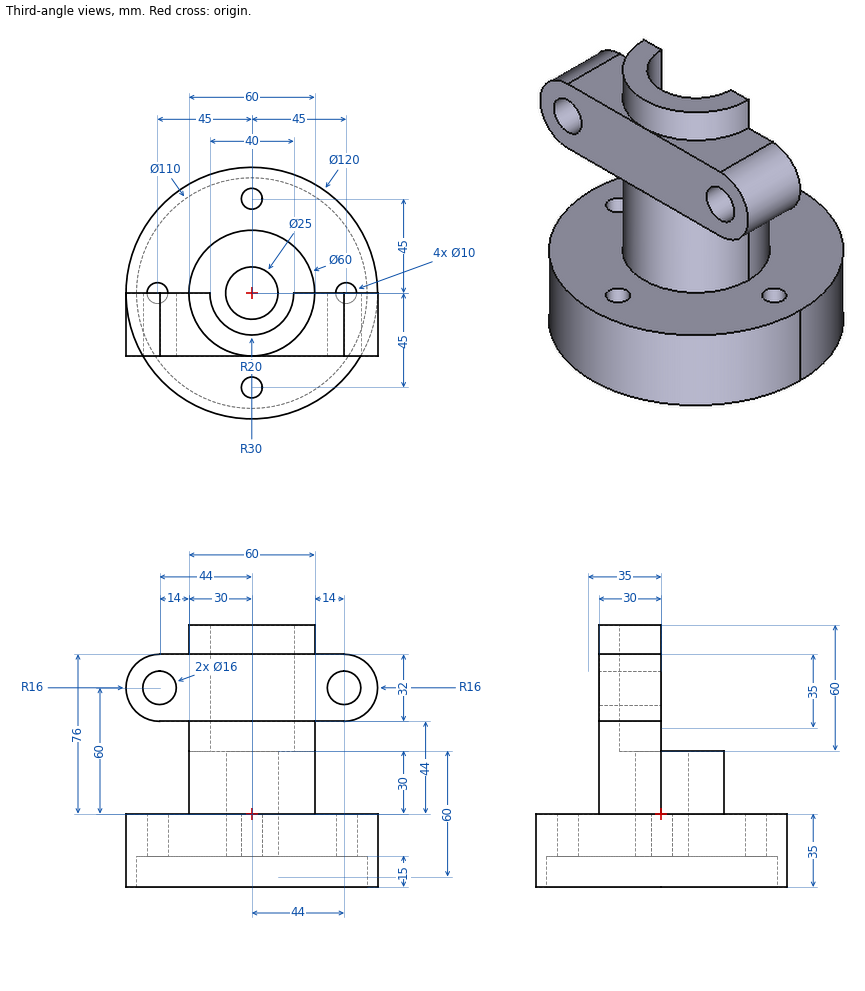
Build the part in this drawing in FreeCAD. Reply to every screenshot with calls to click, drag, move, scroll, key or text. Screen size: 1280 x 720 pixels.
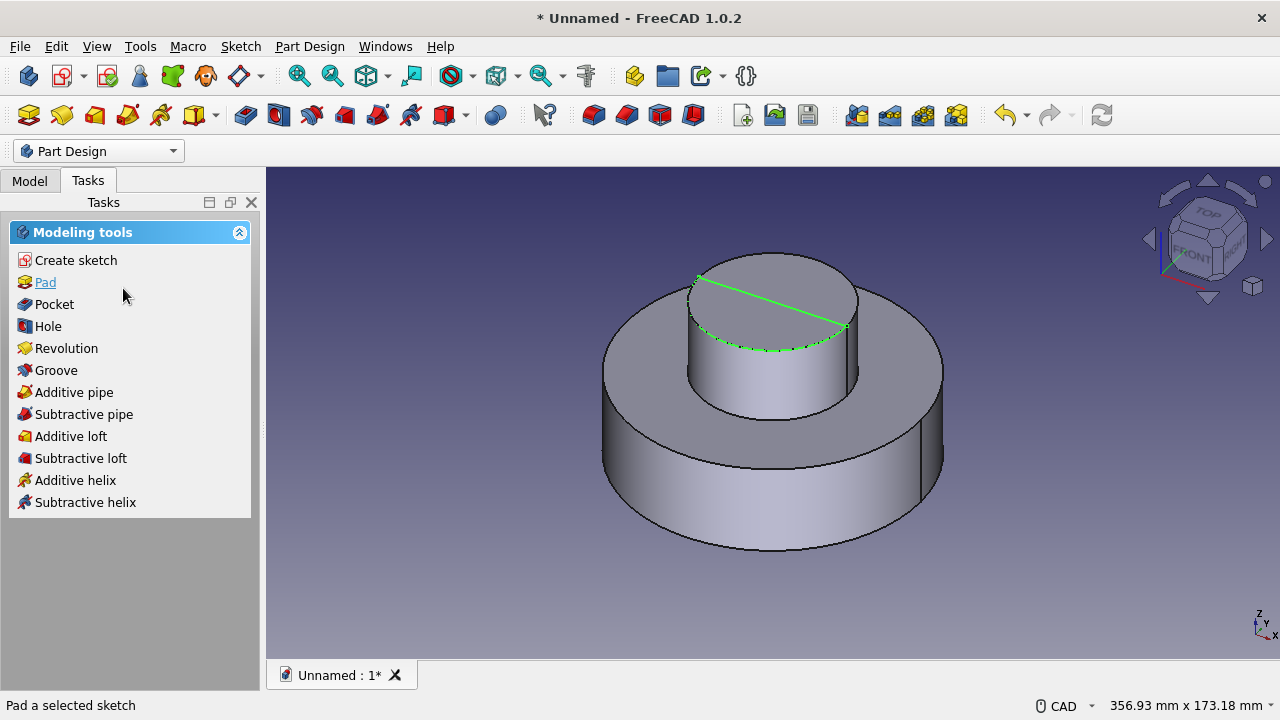
click(29, 116)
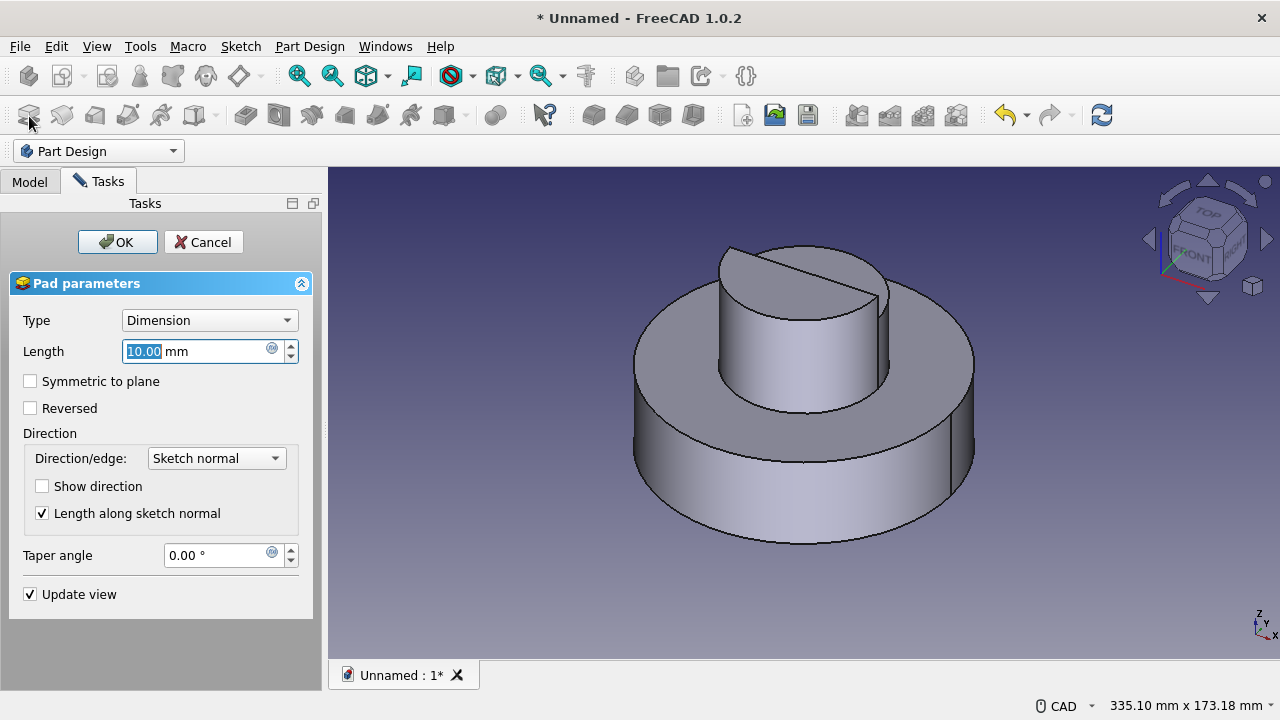
text(60)
key(Tab)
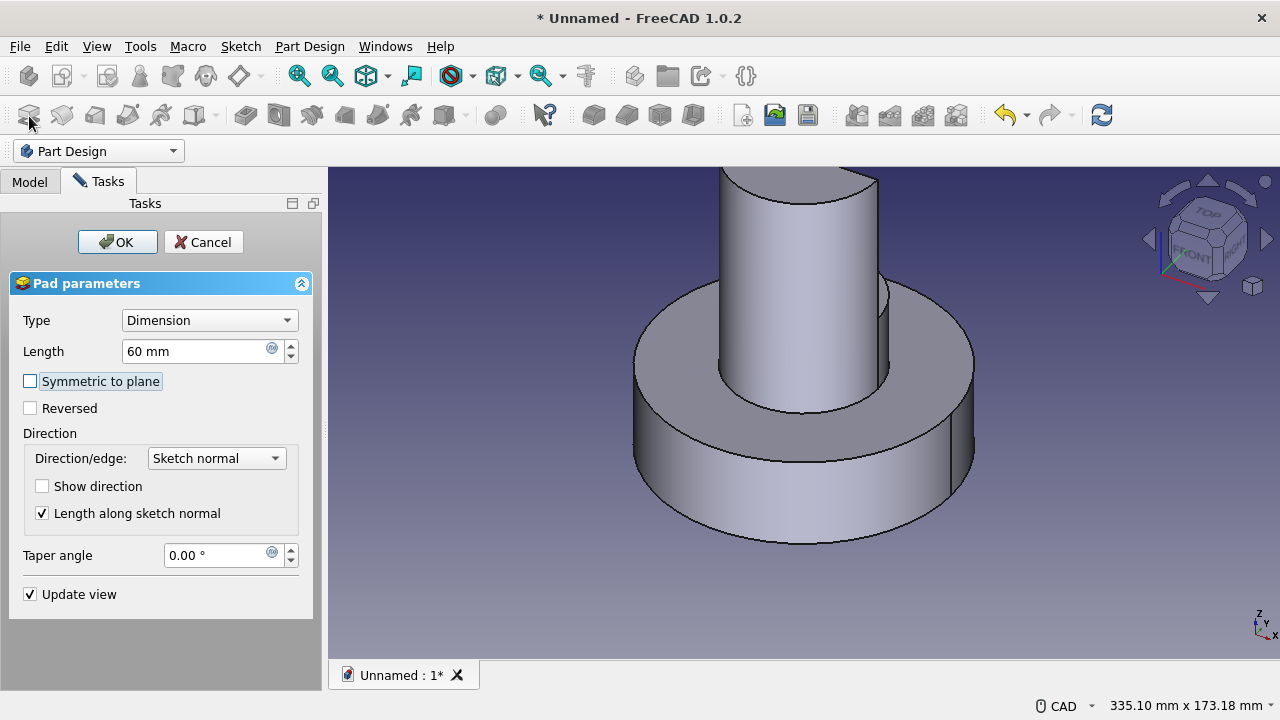
click(118, 242)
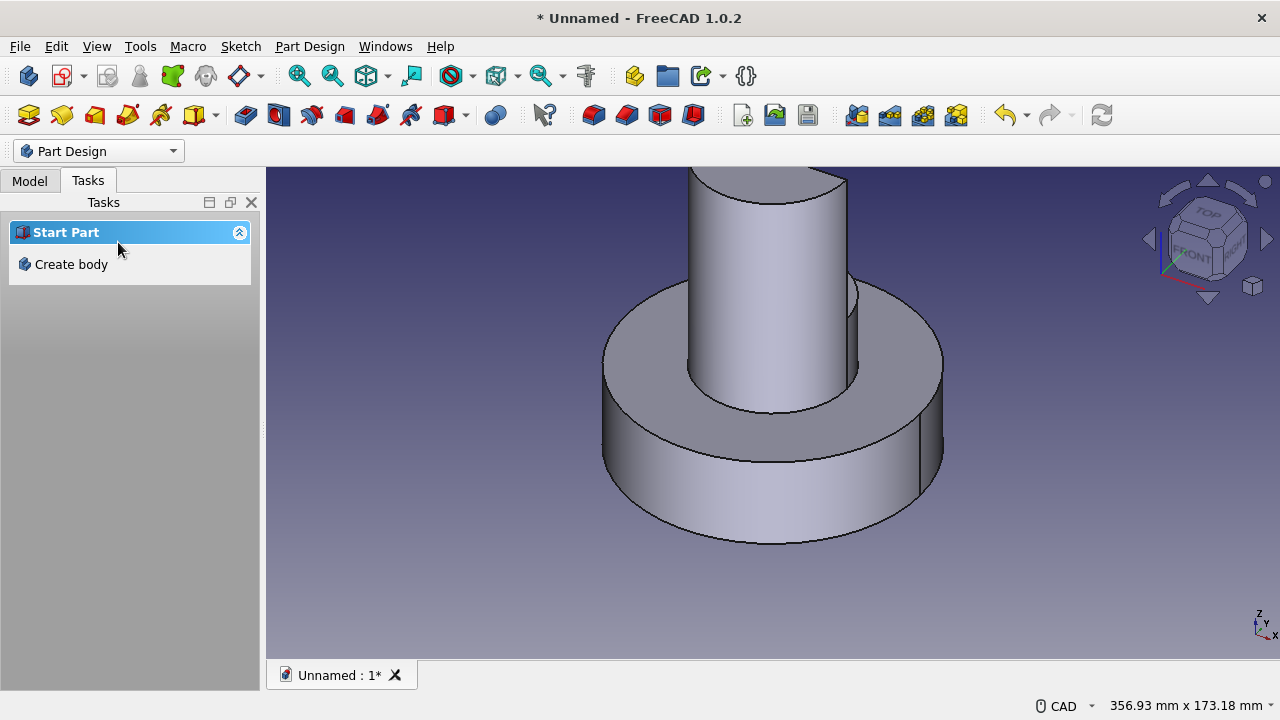
click(300, 76)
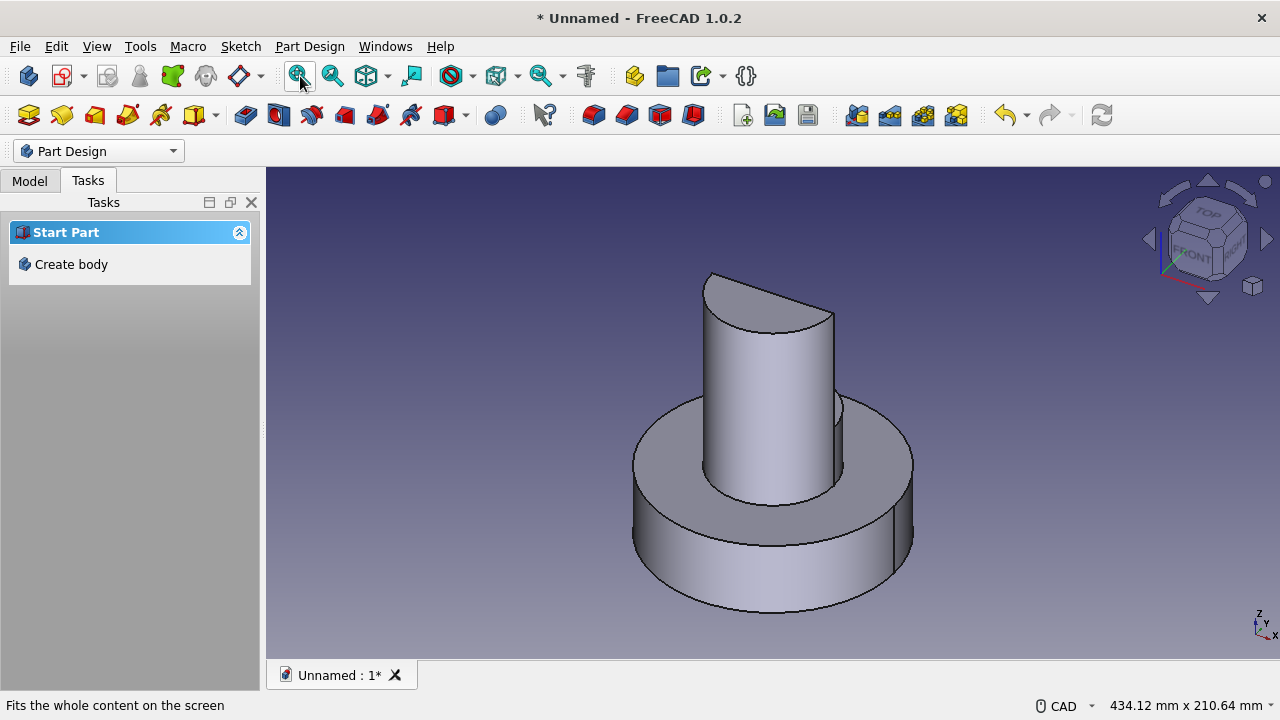
key(5)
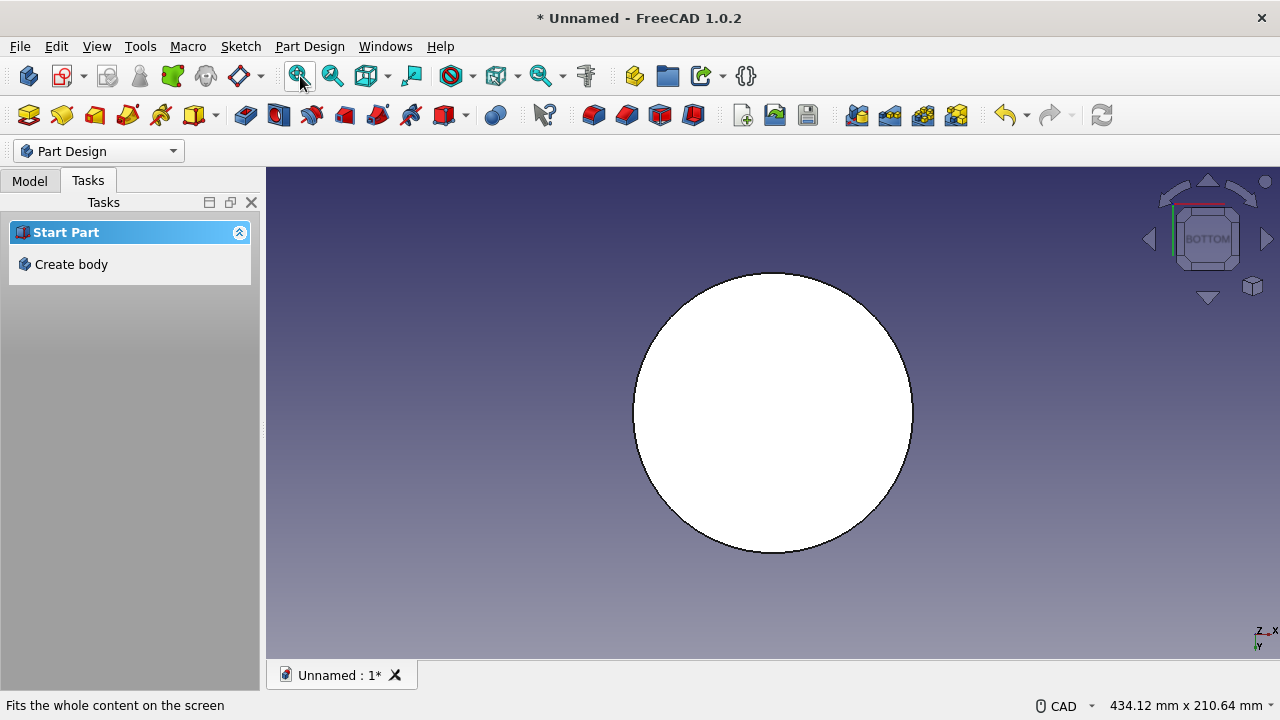
click(773, 412)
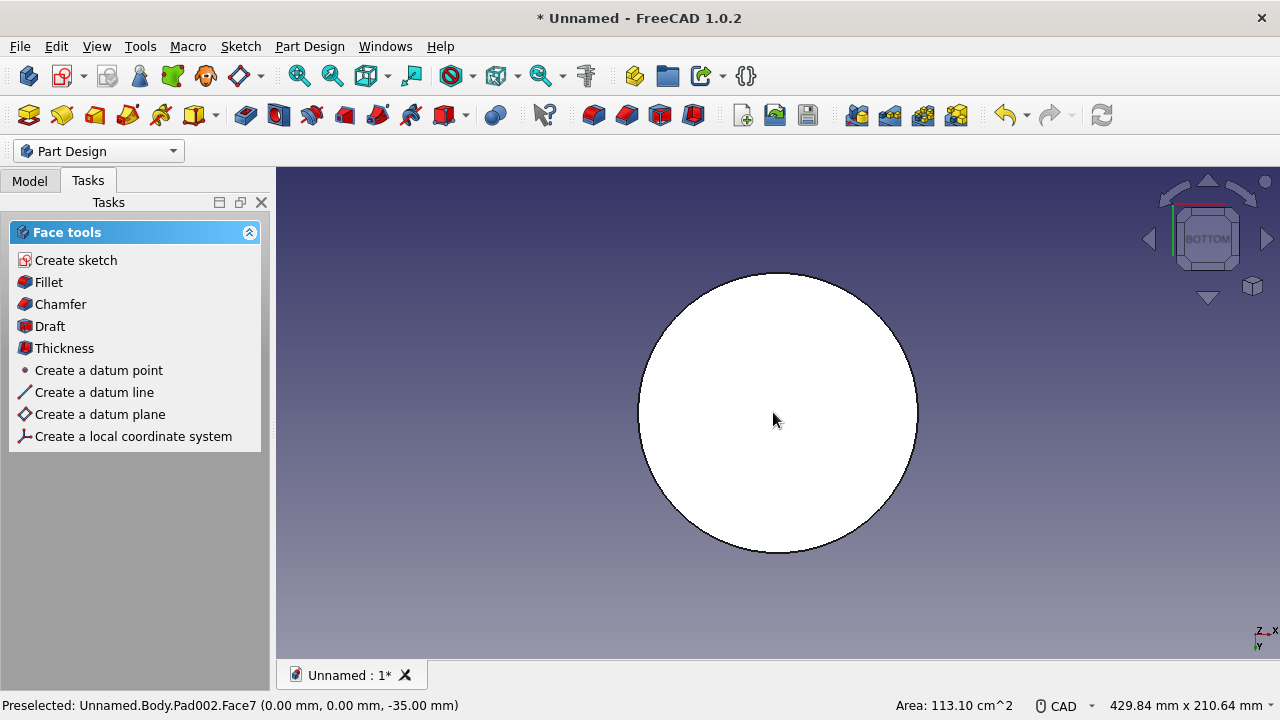
click(62, 76)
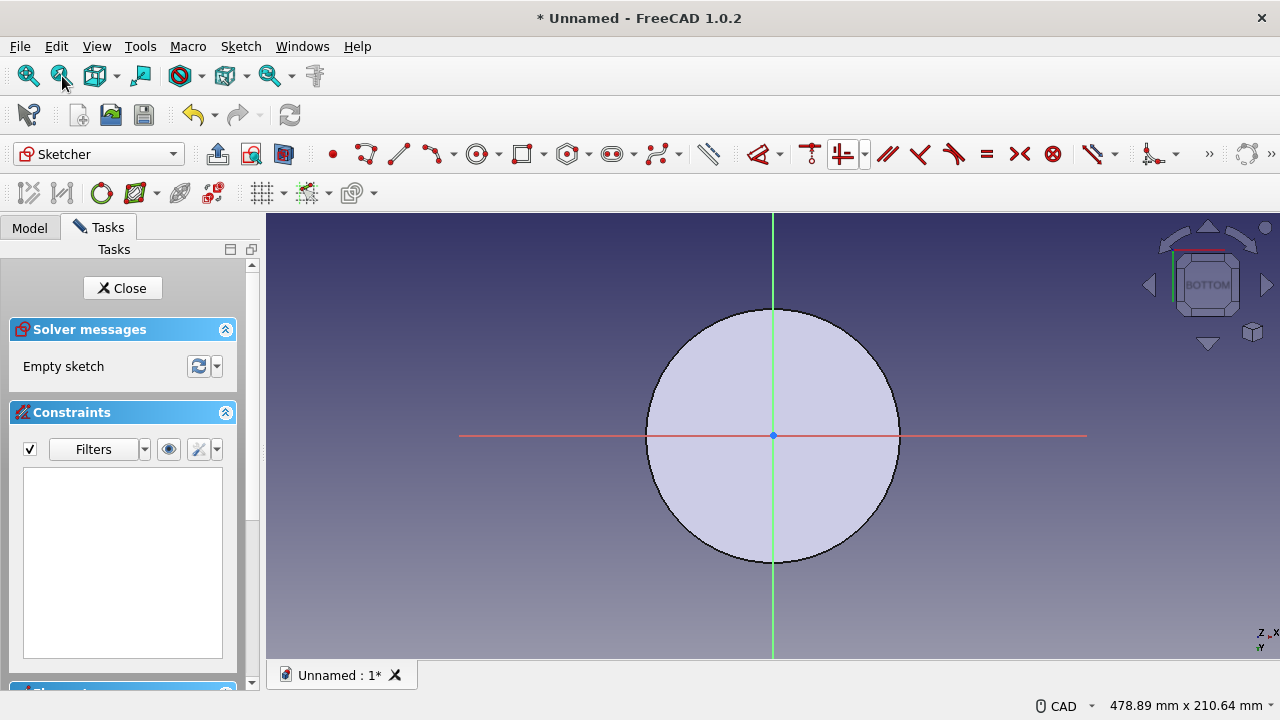
click(476, 154)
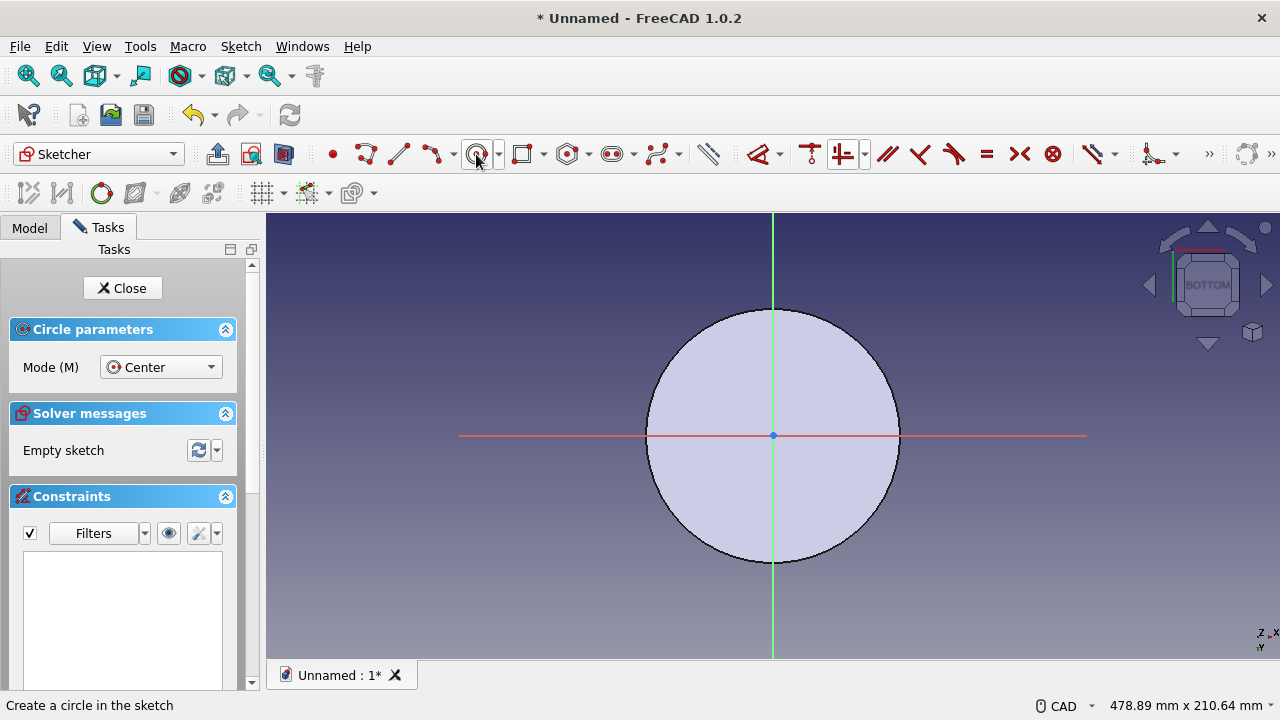
click(773, 436)
move(855, 354)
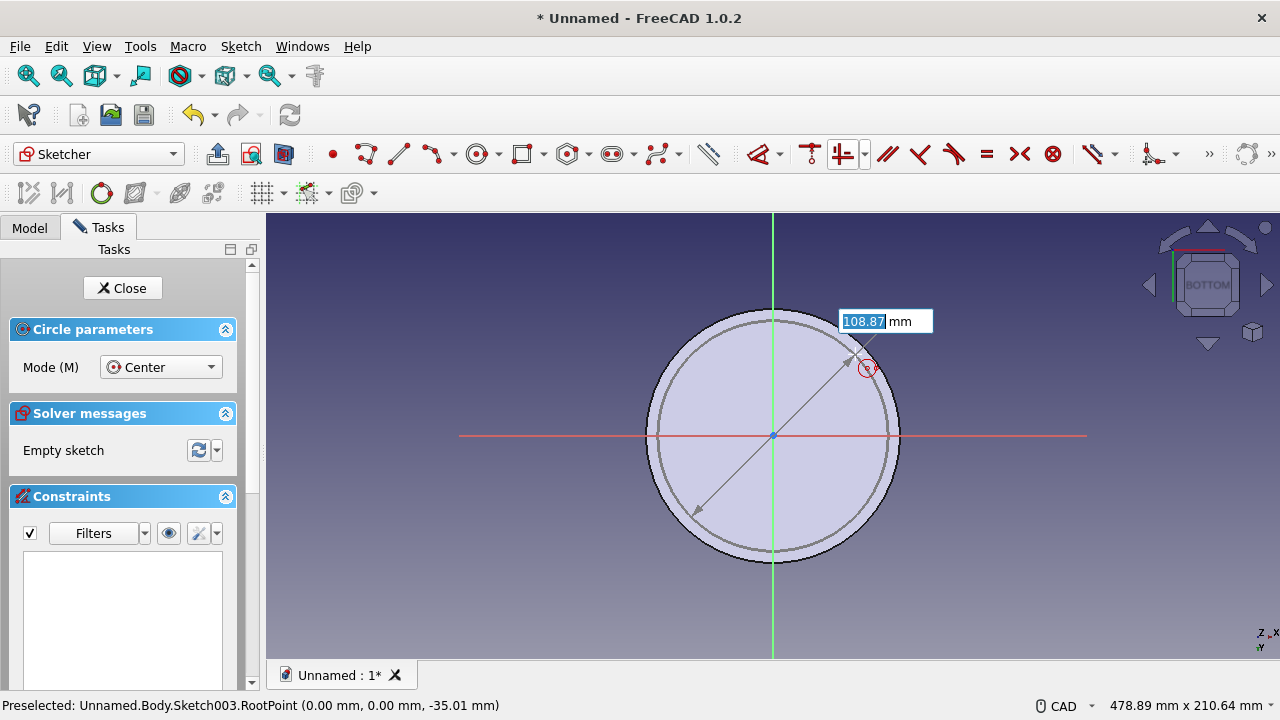
text(110)
key(Return)
key(Escape)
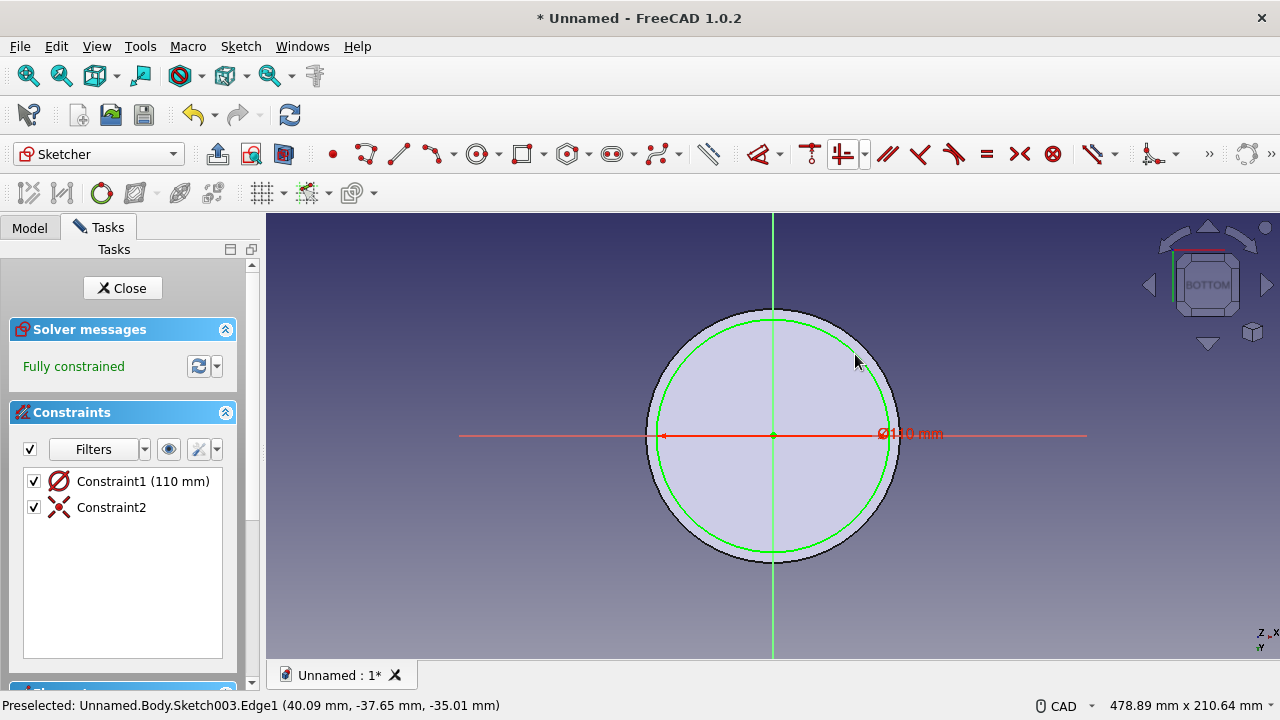
click(123, 288)